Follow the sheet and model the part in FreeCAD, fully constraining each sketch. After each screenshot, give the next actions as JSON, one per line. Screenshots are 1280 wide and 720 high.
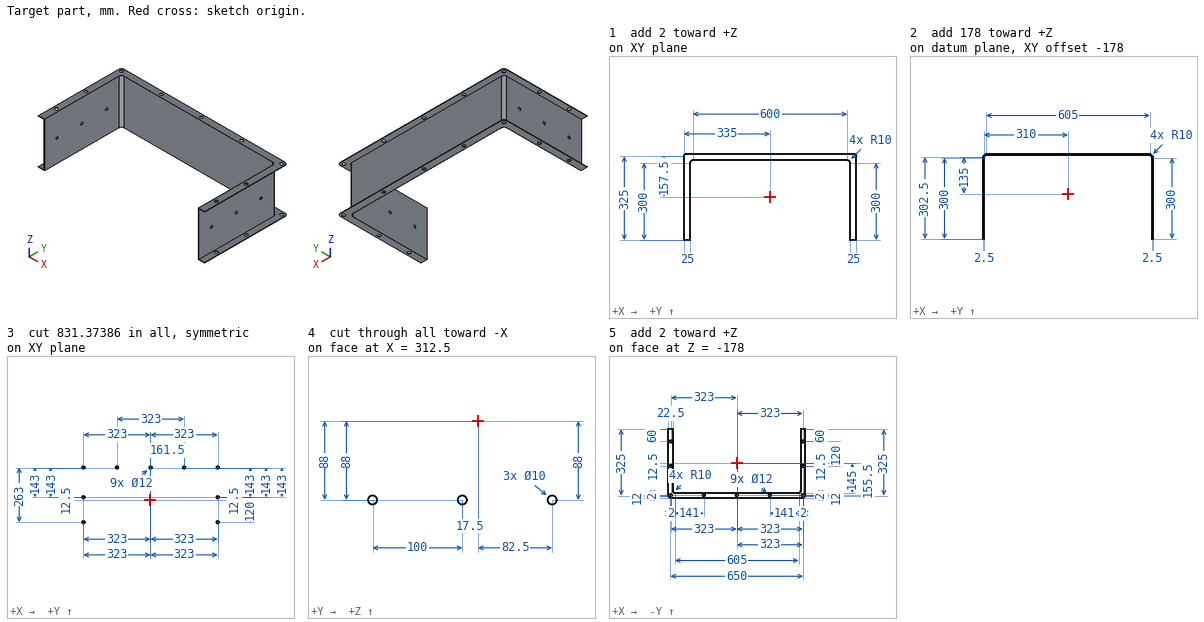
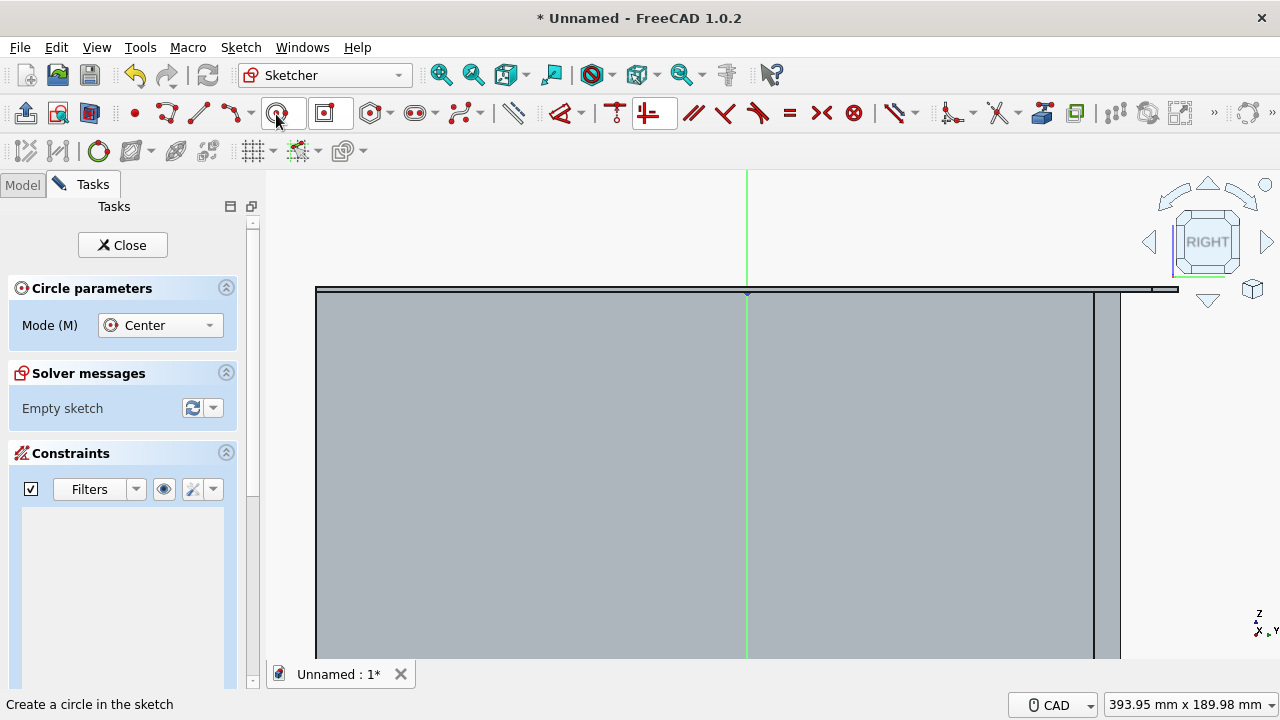
{"action": "scroll", "coordinate": [959, 519], "scroll_direction": "up", "scroll_amount": 3}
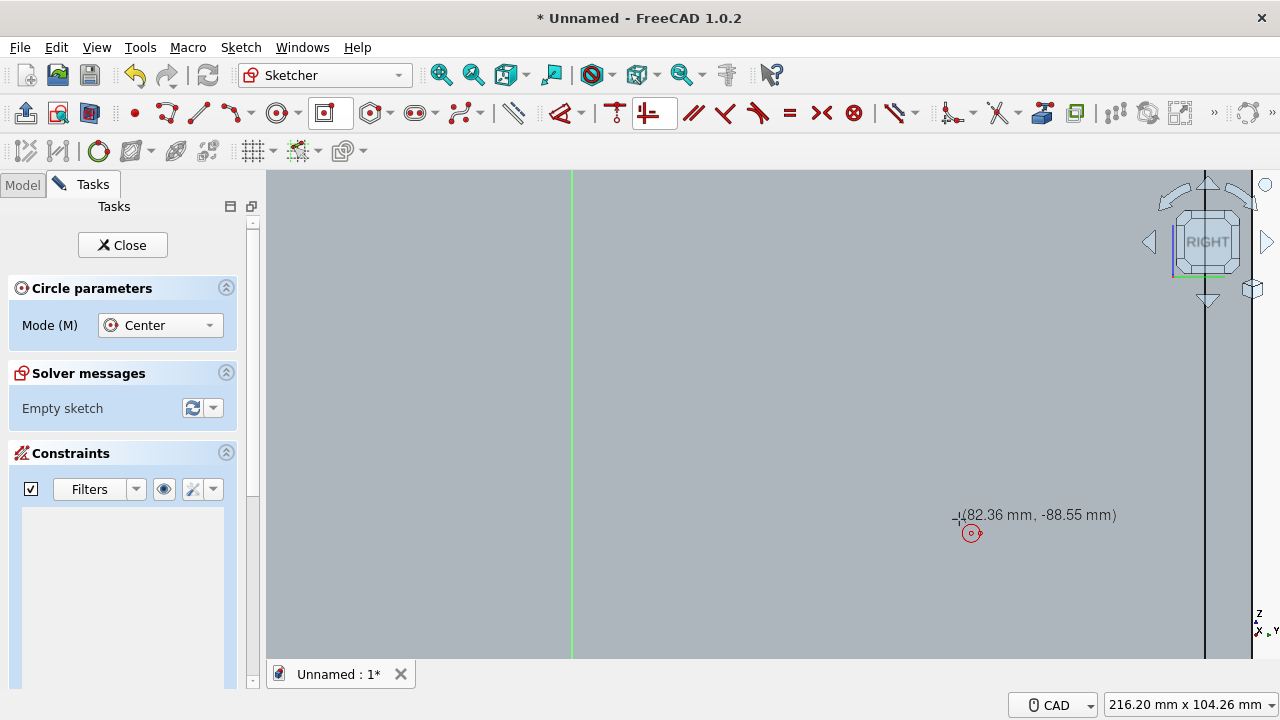
{"action": "left_click", "coordinate": [959, 518]}
{"action": "mouse_move", "coordinate": [976, 501]}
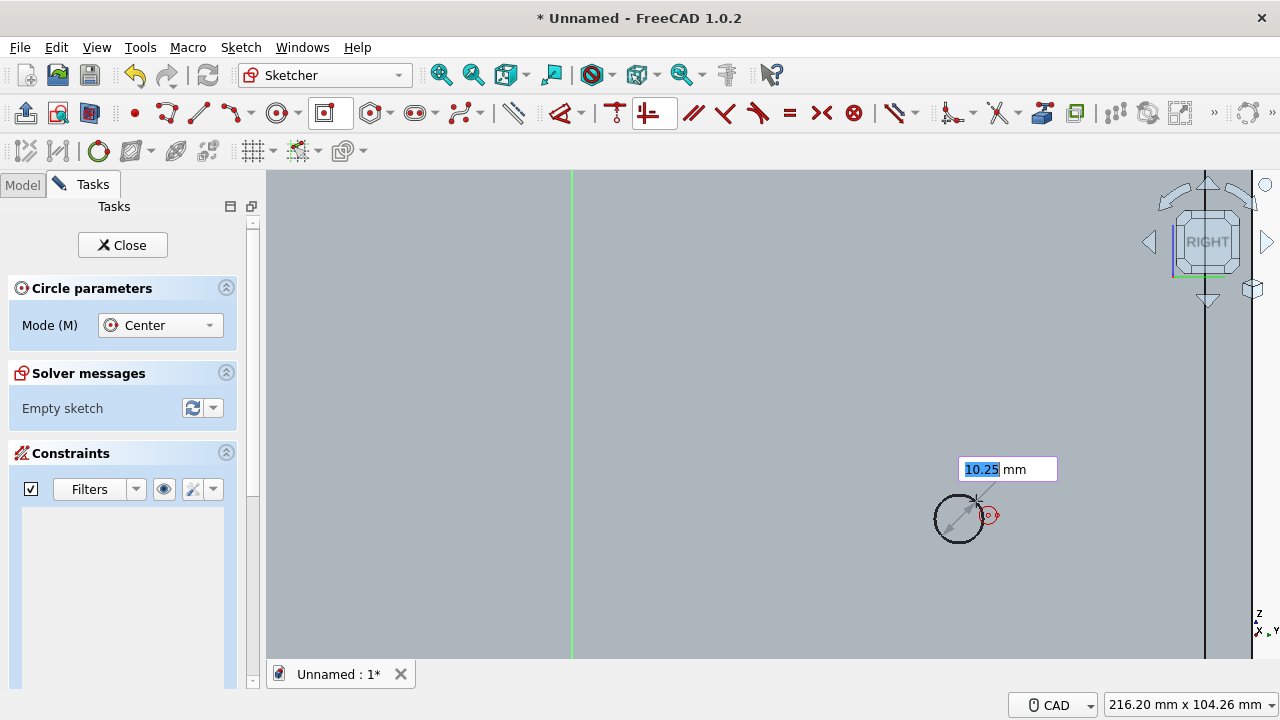
{"action": "type", "text": "10"}
{"action": "key", "text": "Return"}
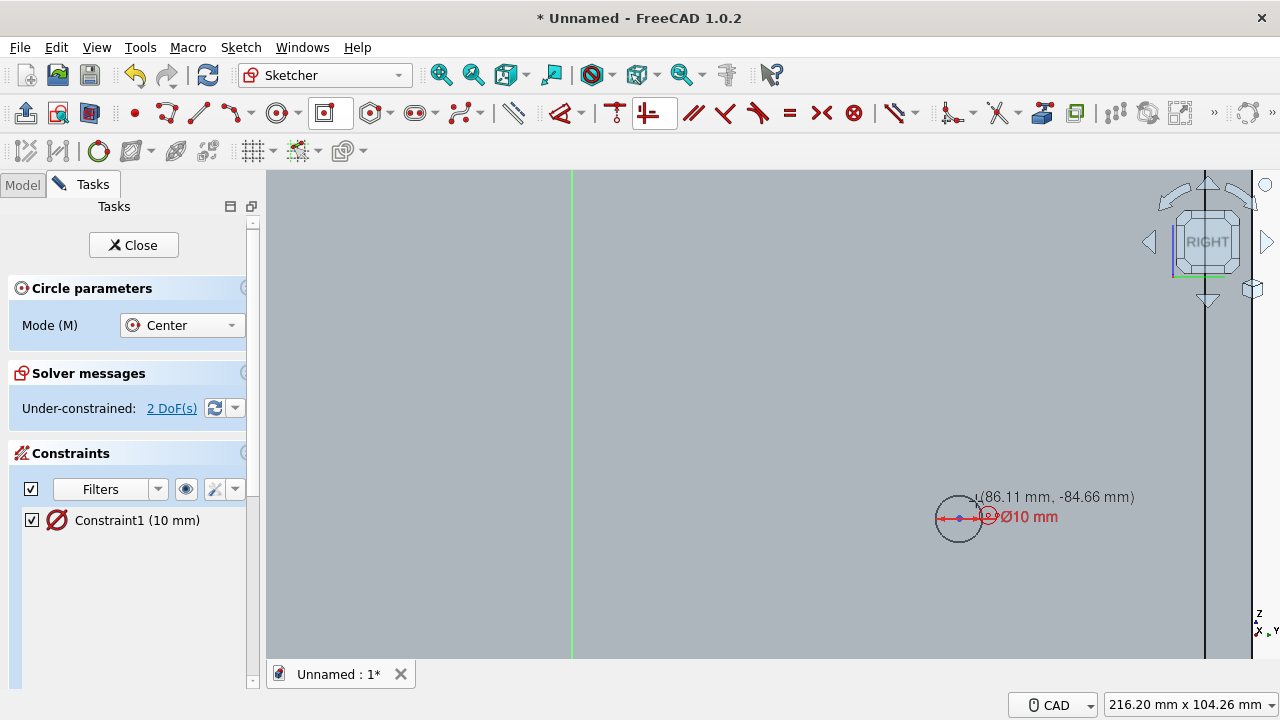
{"action": "left_click", "coordinate": [490, 518]}
{"action": "mouse_move", "coordinate": [507, 501]}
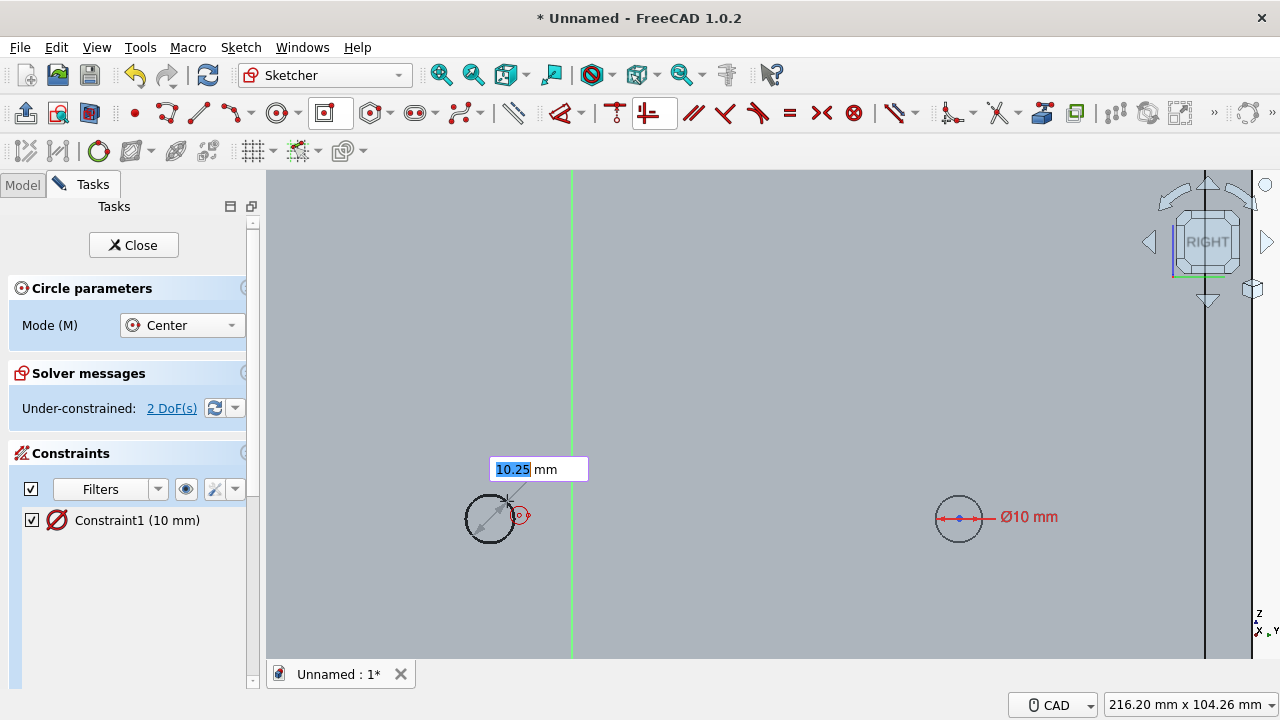
{"action": "type", "text": "10"}
{"action": "key", "text": "Return"}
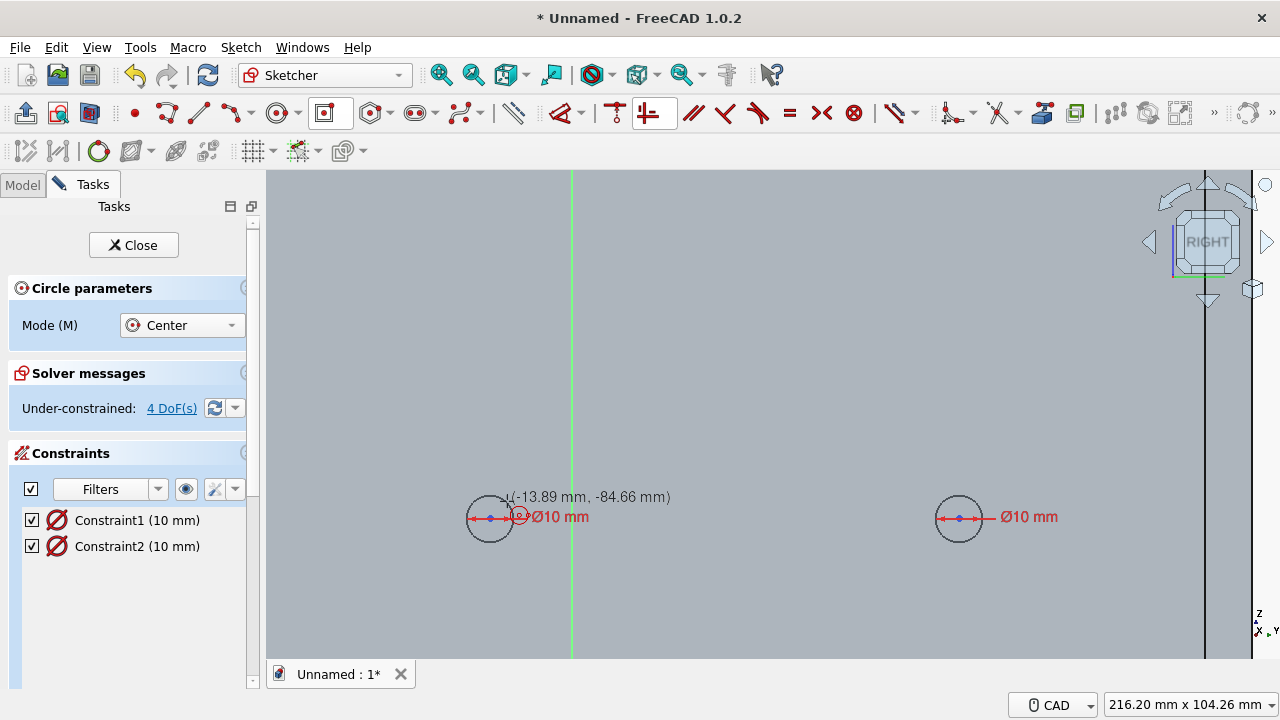
{"action": "scroll", "coordinate": [965, 526], "scroll_direction": "down", "scroll_amount": 3}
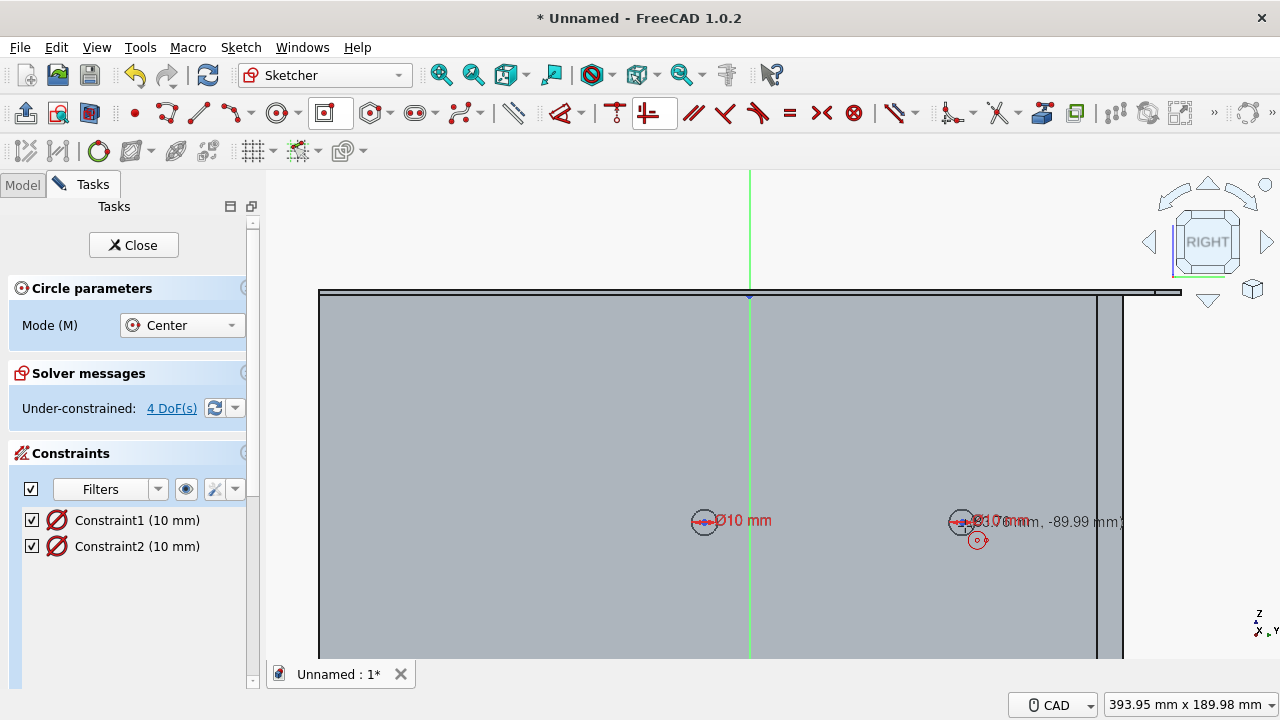
{"action": "scroll", "coordinate": [447, 522], "scroll_direction": "up", "scroll_amount": 3}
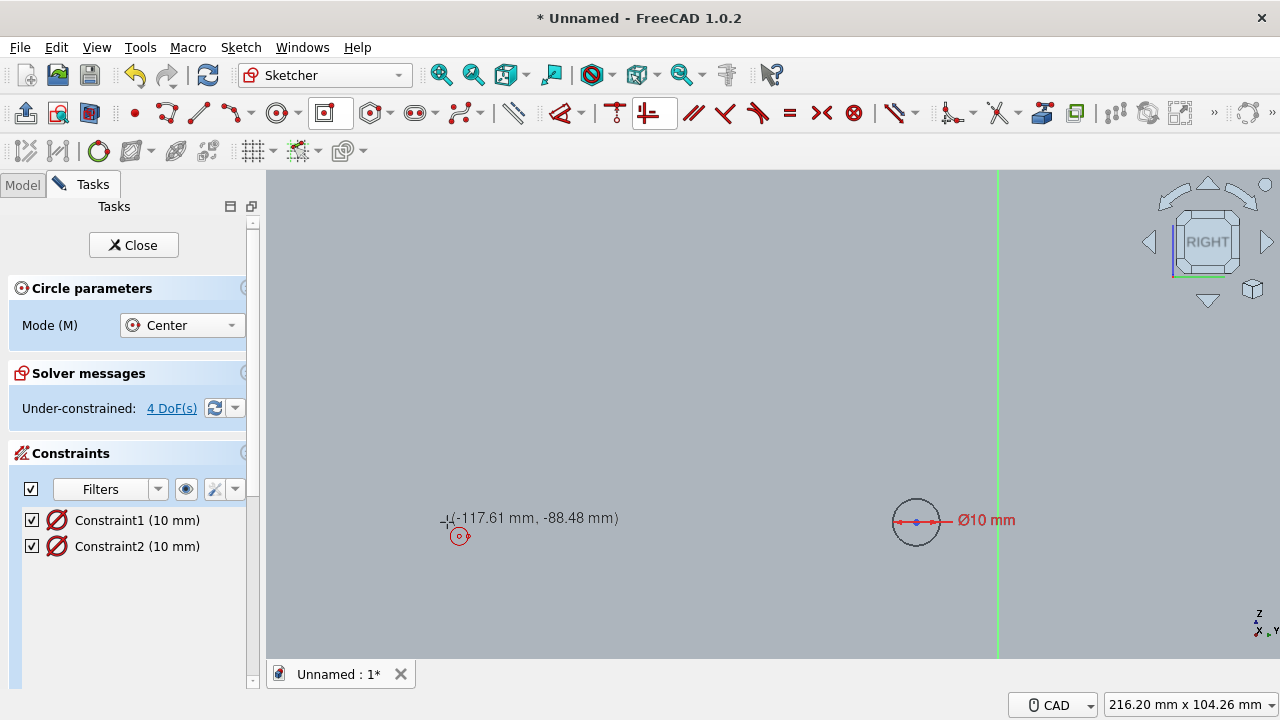
{"action": "left_click", "coordinate": [447, 521]}
{"action": "mouse_move", "coordinate": [464, 504]}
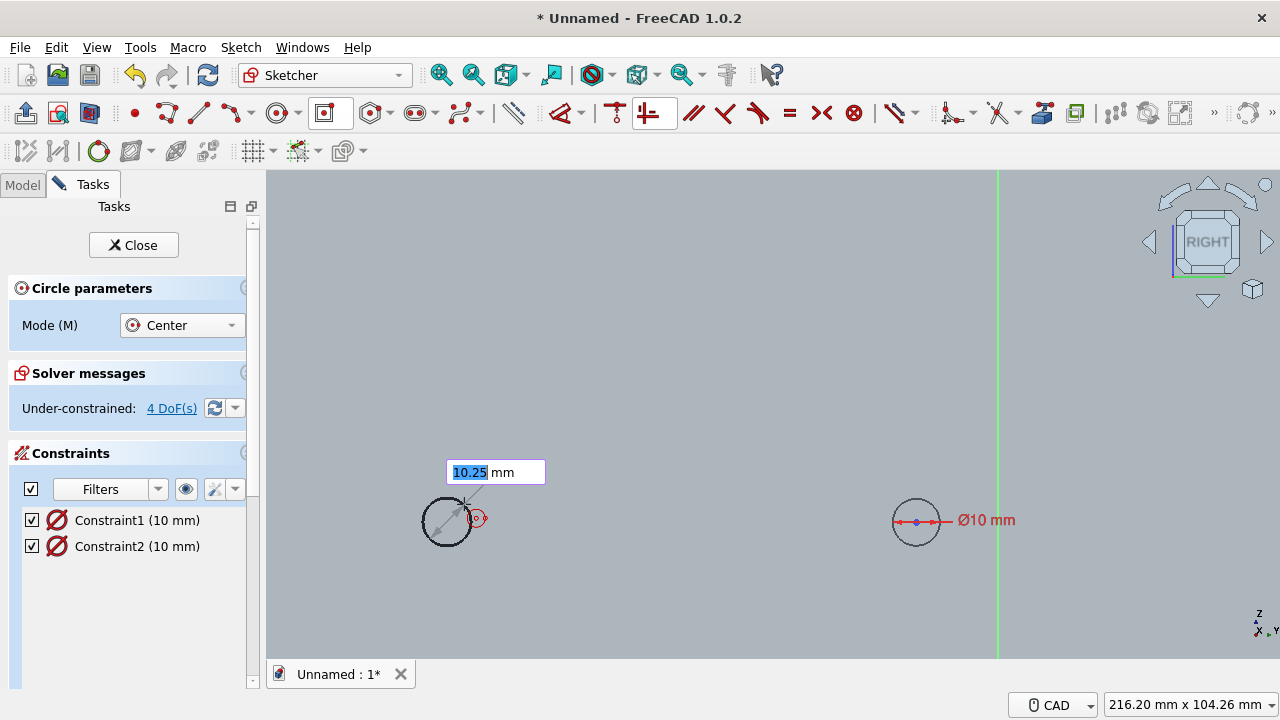
{"action": "type", "text": "10"}
{"action": "key", "text": "Return"}
{"action": "key", "text": "Escape"}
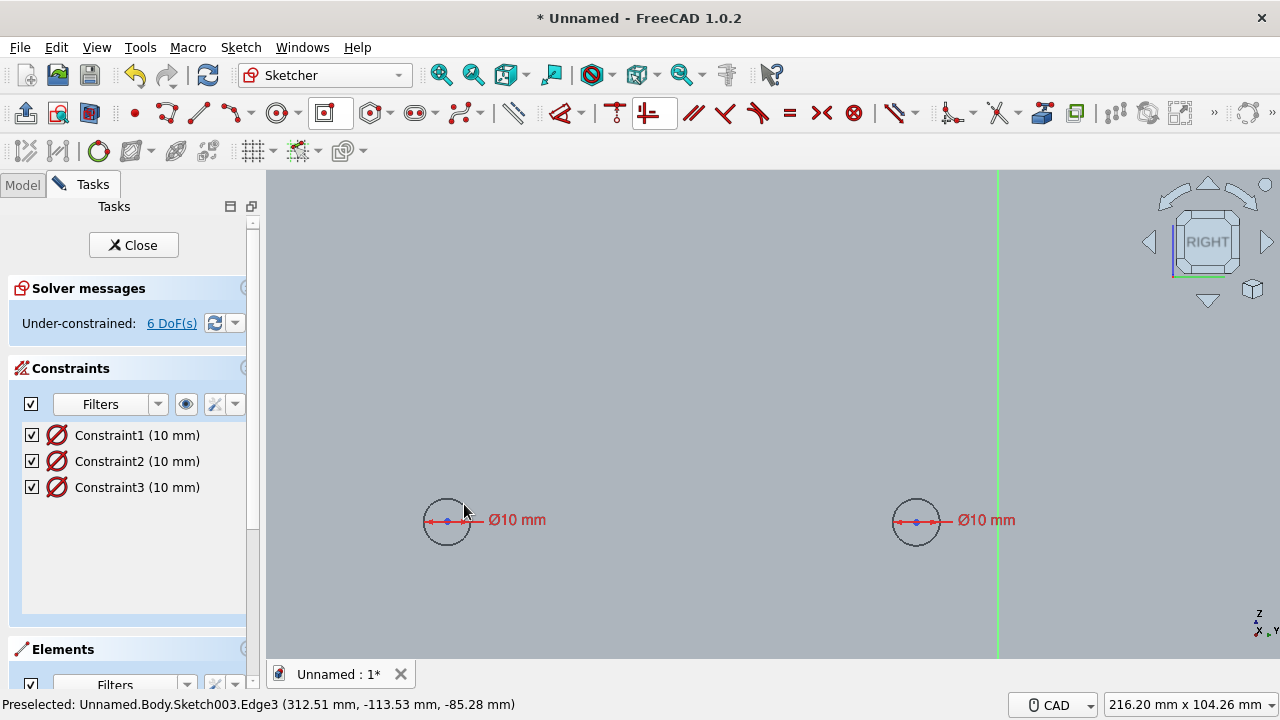
{"action": "left_click", "coordinate": [560, 114]}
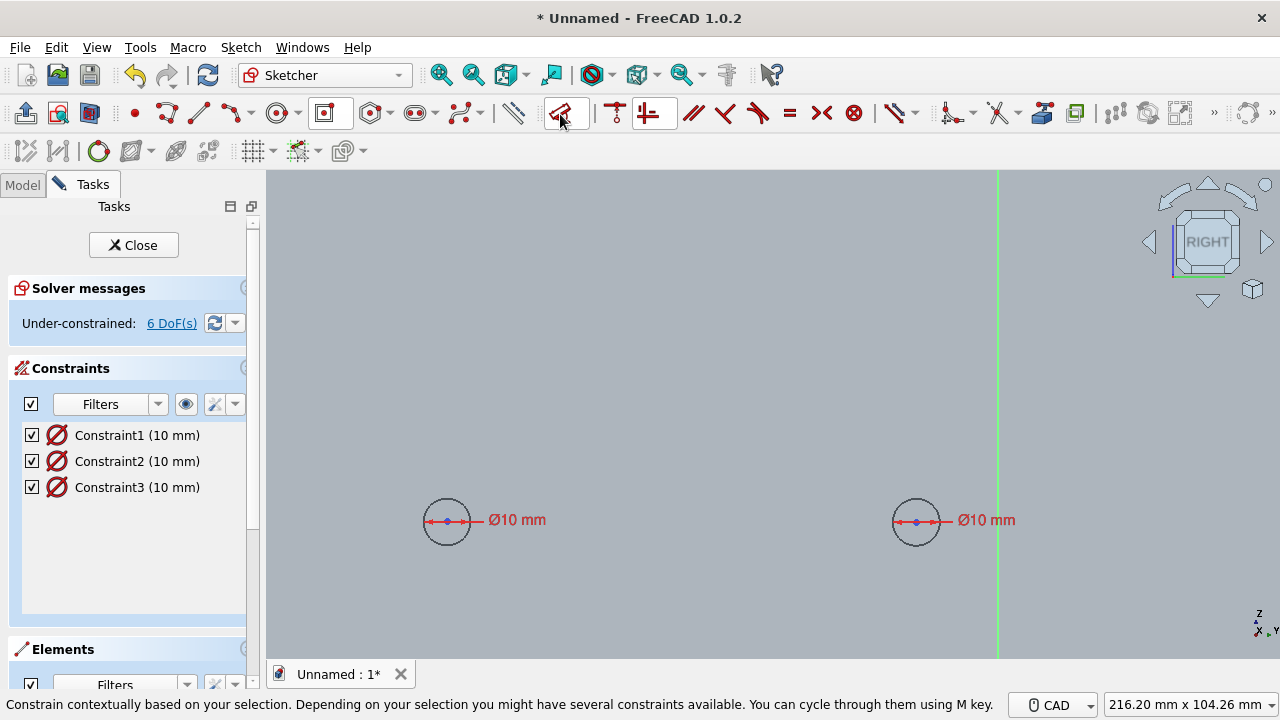
{"action": "scroll", "coordinate": [447, 522], "scroll_direction": "down", "scroll_amount": 3}